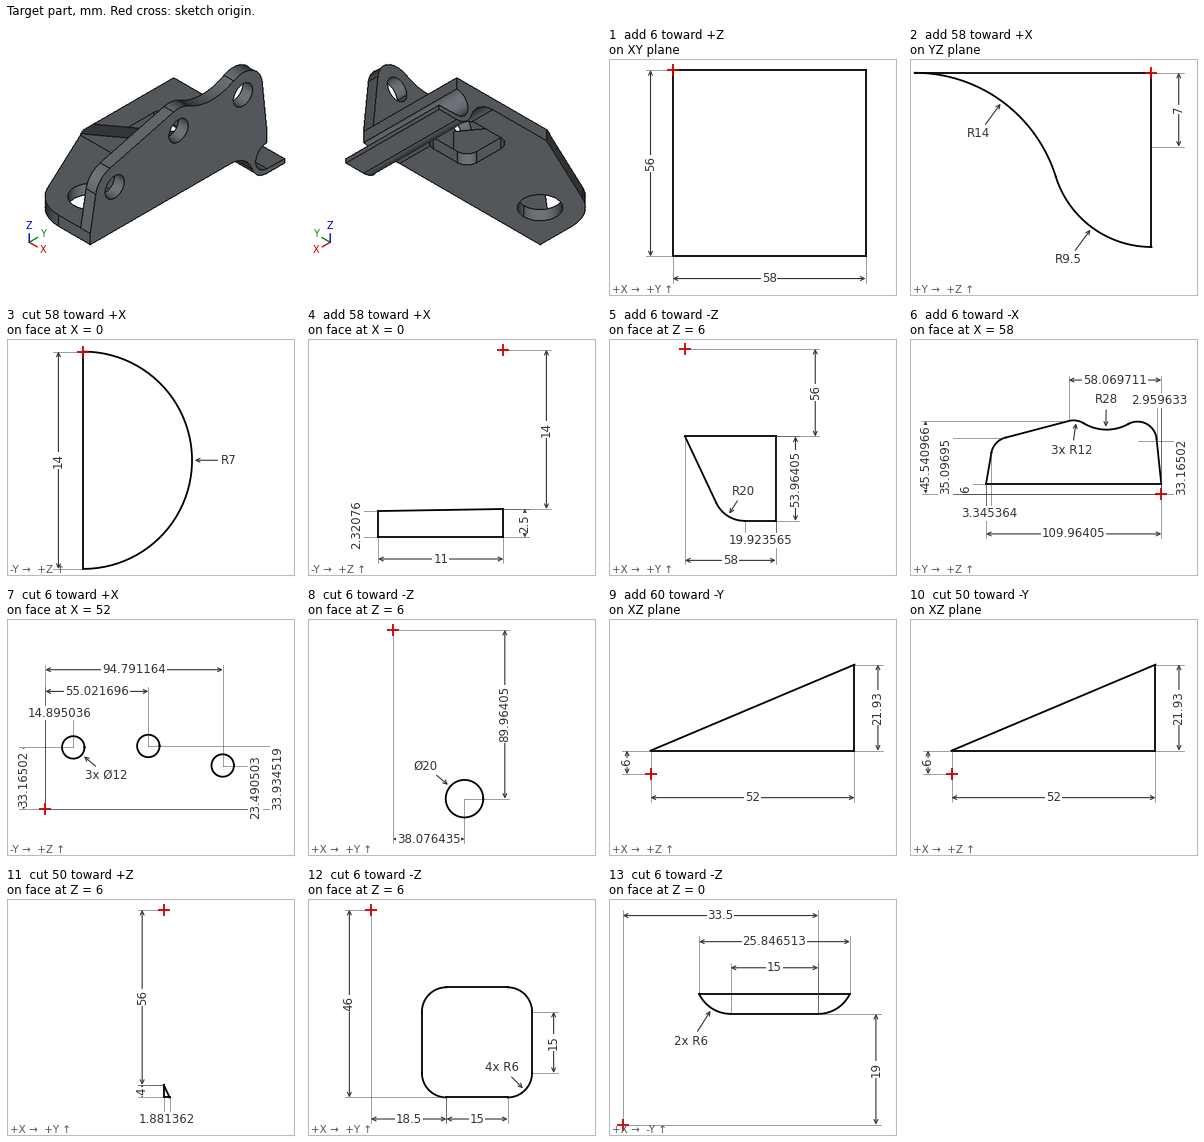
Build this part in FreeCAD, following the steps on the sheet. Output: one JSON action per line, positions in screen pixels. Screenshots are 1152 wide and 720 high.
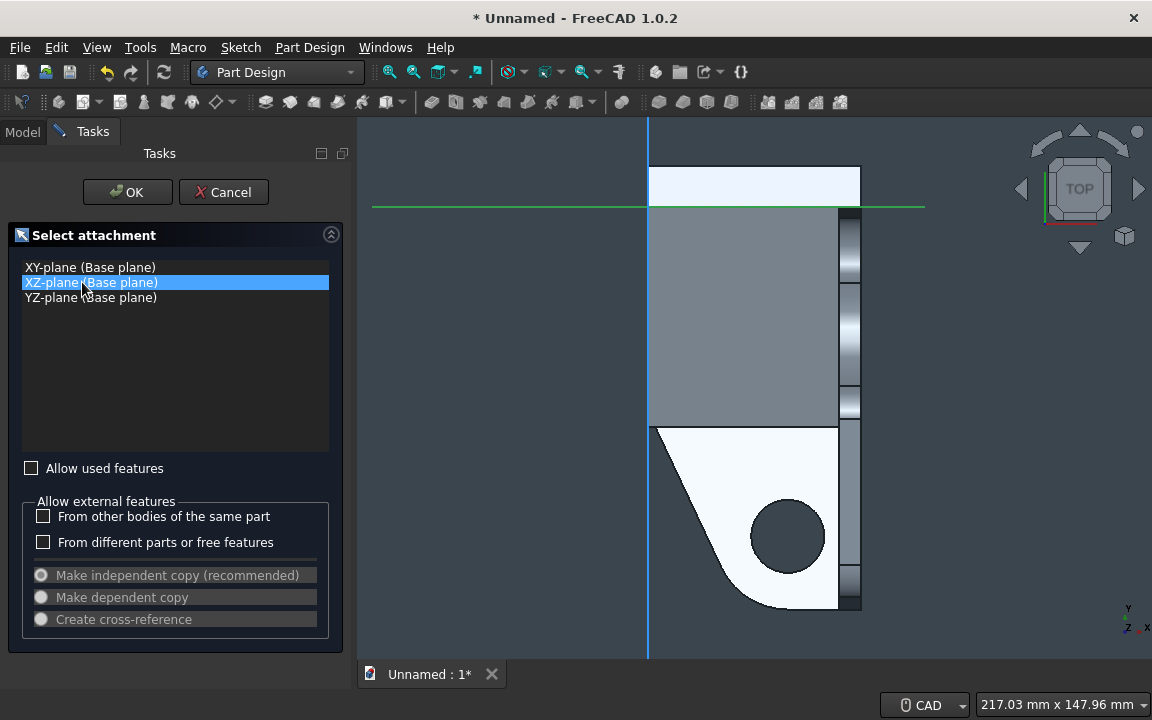
{"action": "left_click", "coordinate": [128, 192]}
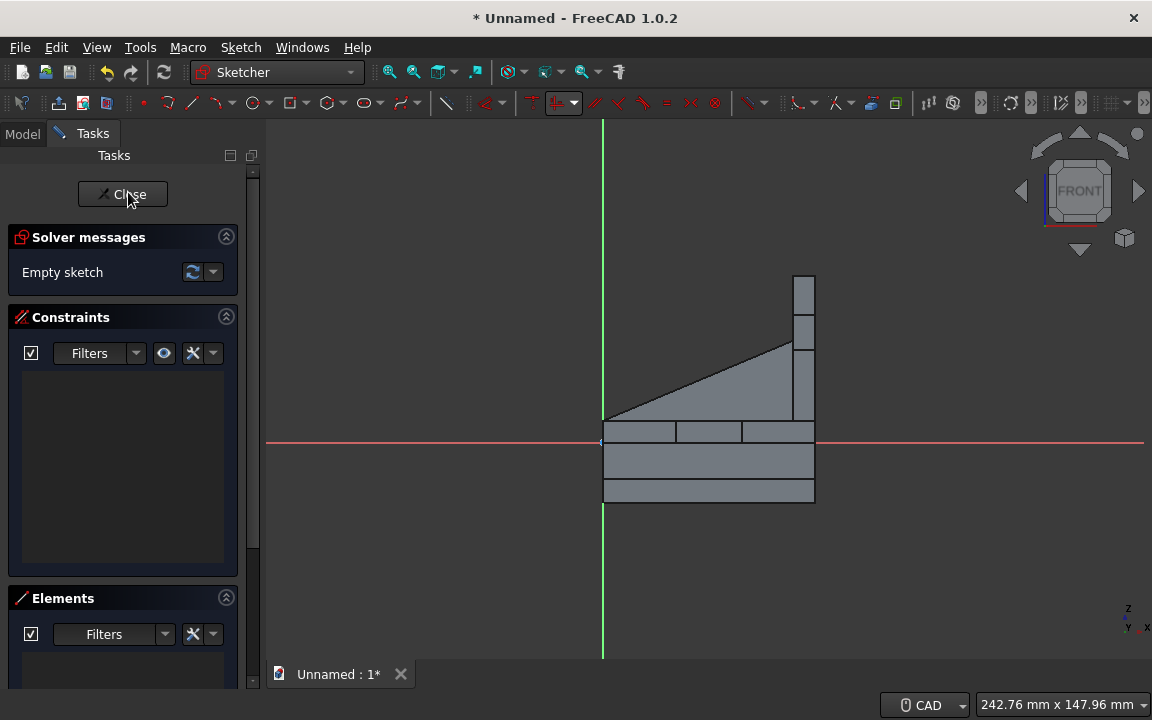
{"action": "left_click", "coordinate": [108, 104]}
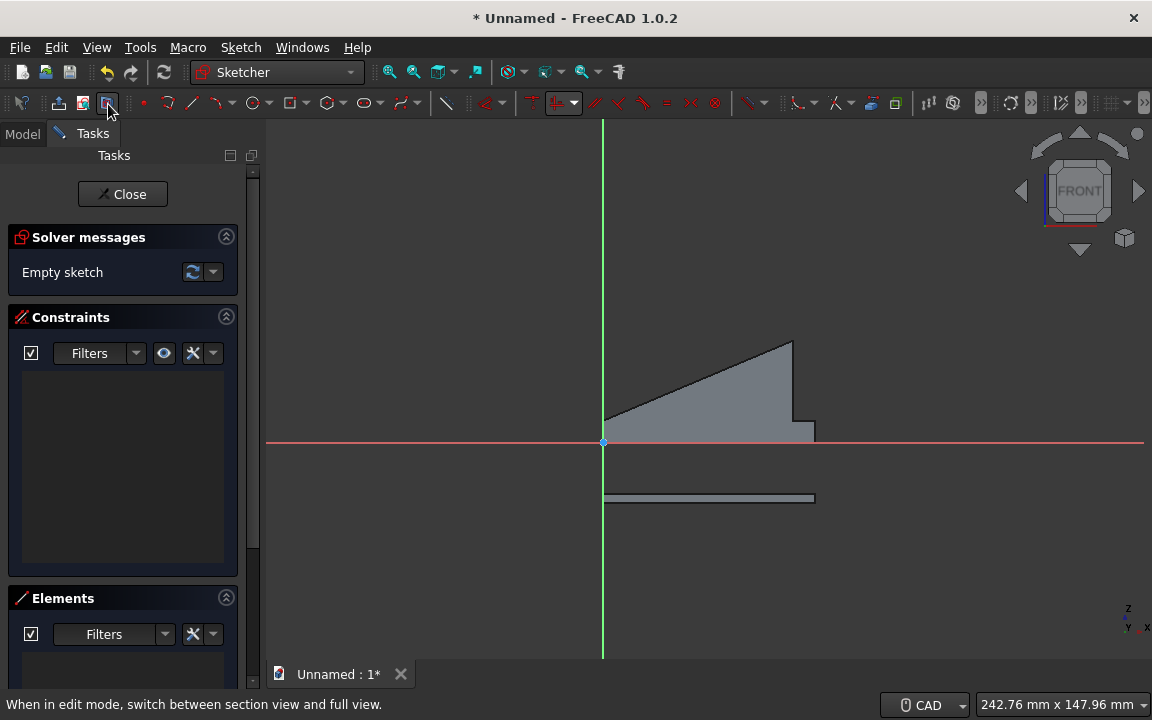
{"action": "scroll", "coordinate": [732, 393], "scroll_direction": "up", "scroll_amount": 5}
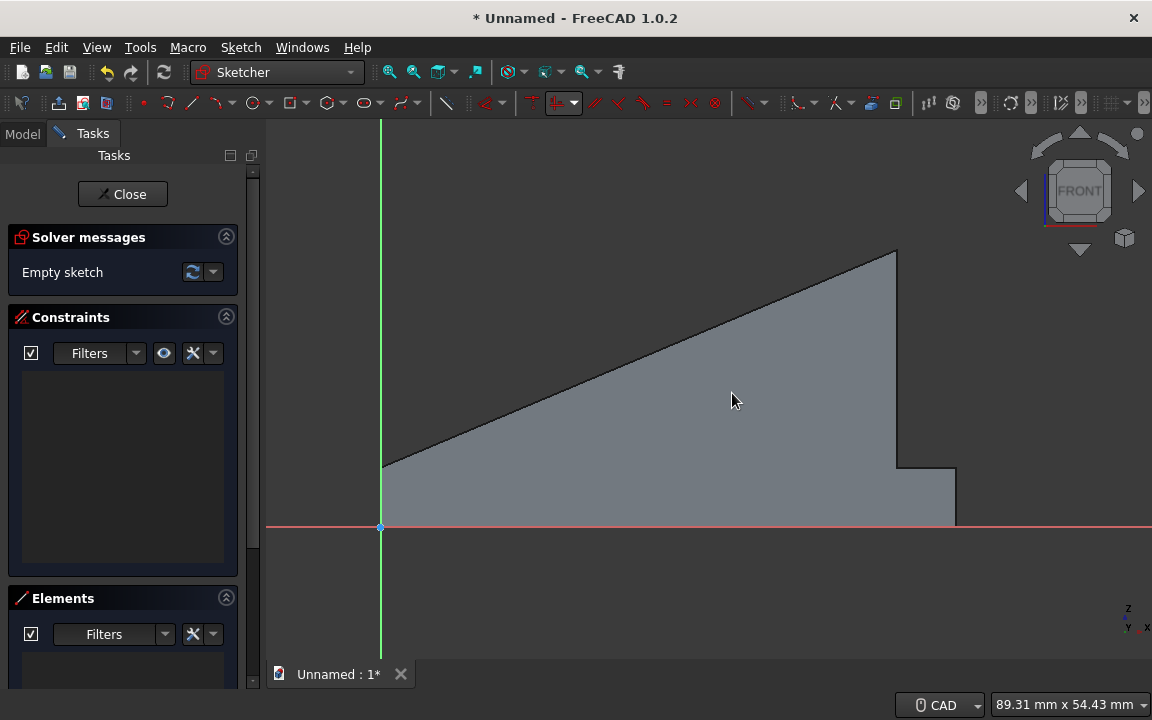
{"action": "left_click", "coordinate": [168, 104]}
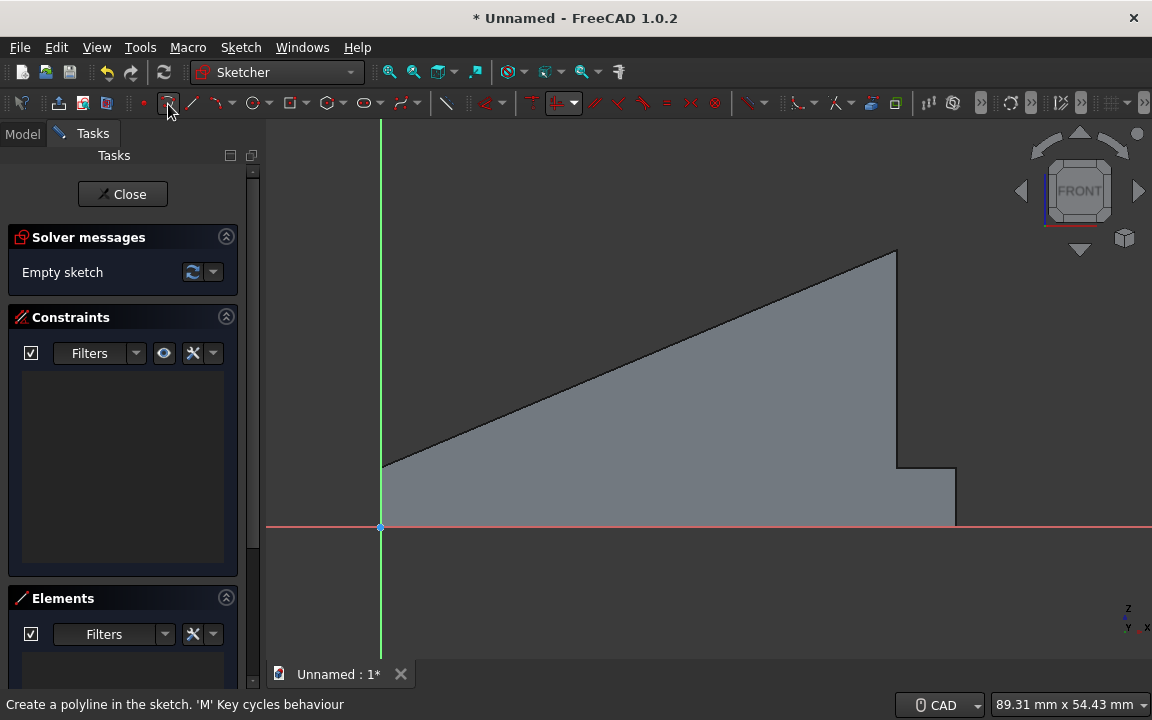
{"action": "left_click", "coordinate": [381, 468]}
{"action": "left_click", "coordinate": [897, 250]}
{"action": "left_click", "coordinate": [897, 468]}
{"action": "left_click", "coordinate": [381, 469]}
{"action": "key", "text": "Escape"}
{"action": "key", "text": "Escape"}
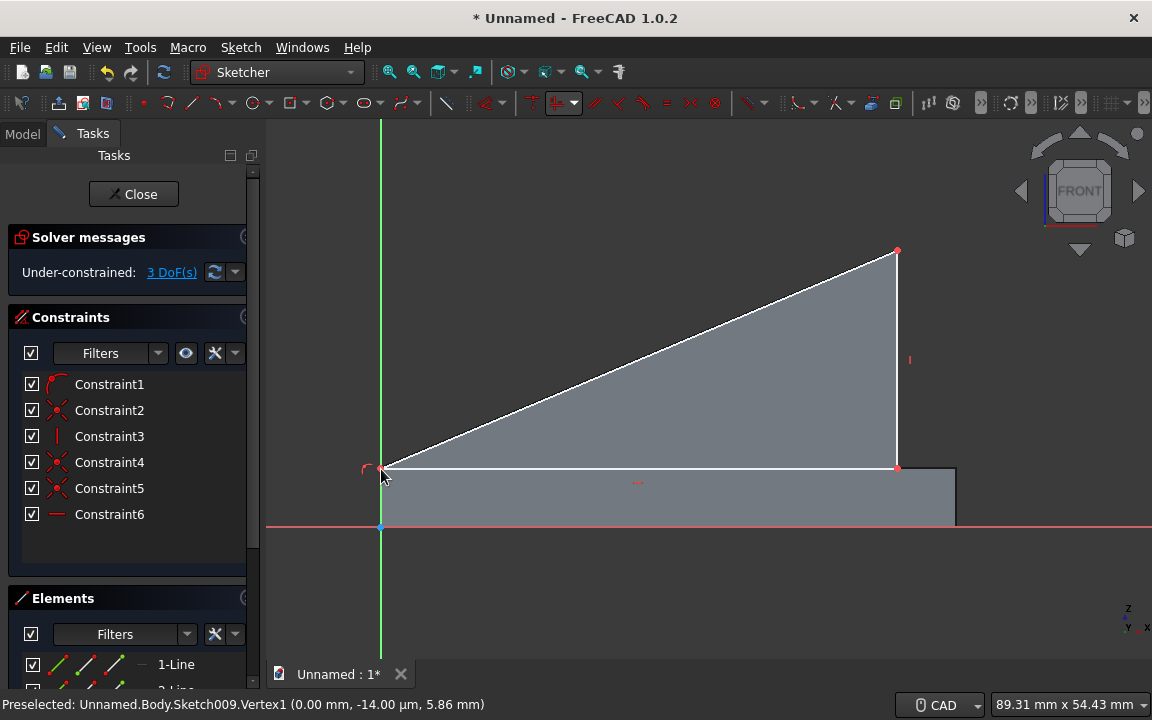
{"action": "left_click", "coordinate": [486, 104]}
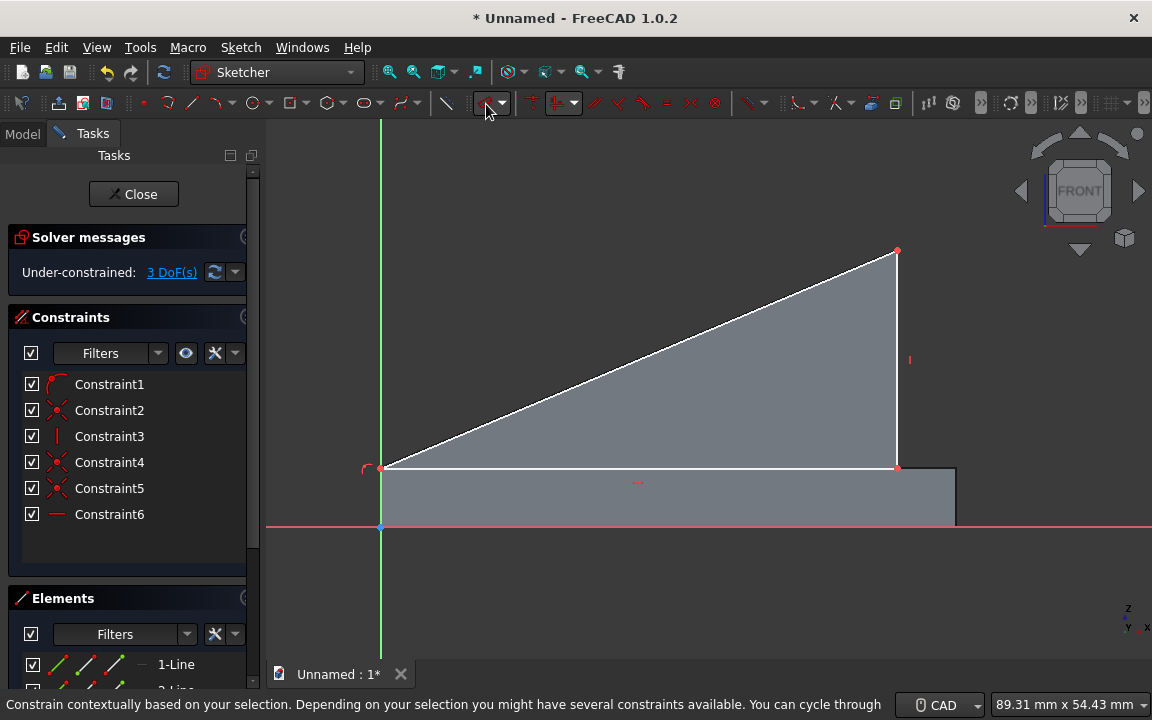
{"action": "left_click", "coordinate": [742, 469]}
{"action": "left_click", "coordinate": [639, 503]}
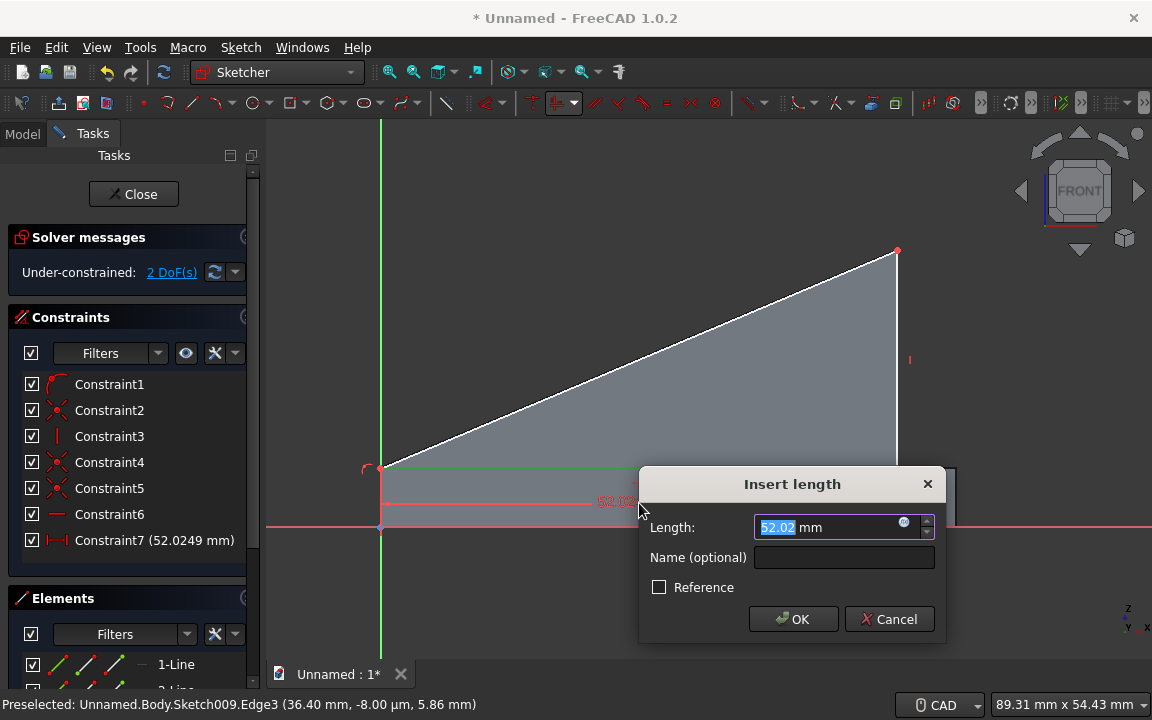
{"action": "type", "text": "52"}
{"action": "key", "text": "Return"}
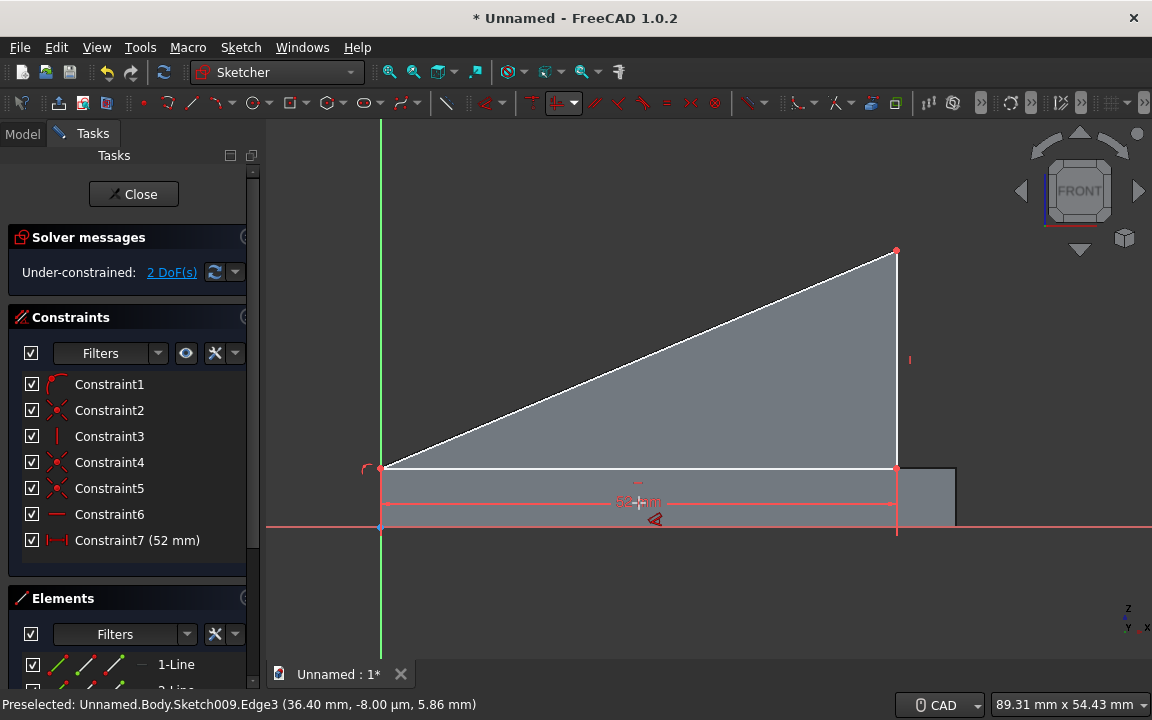
{"action": "left_click", "coordinate": [381, 469]}
{"action": "left_click", "coordinate": [347, 498]}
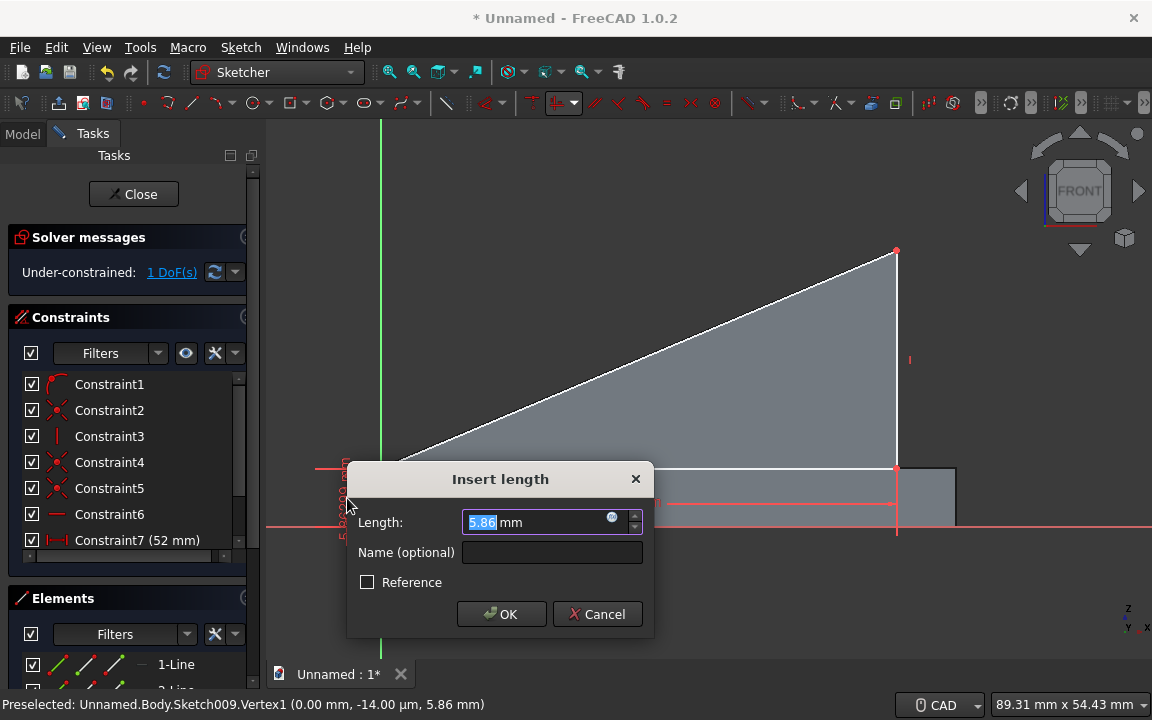
{"action": "type", "text": "6"}
{"action": "key", "text": "Return"}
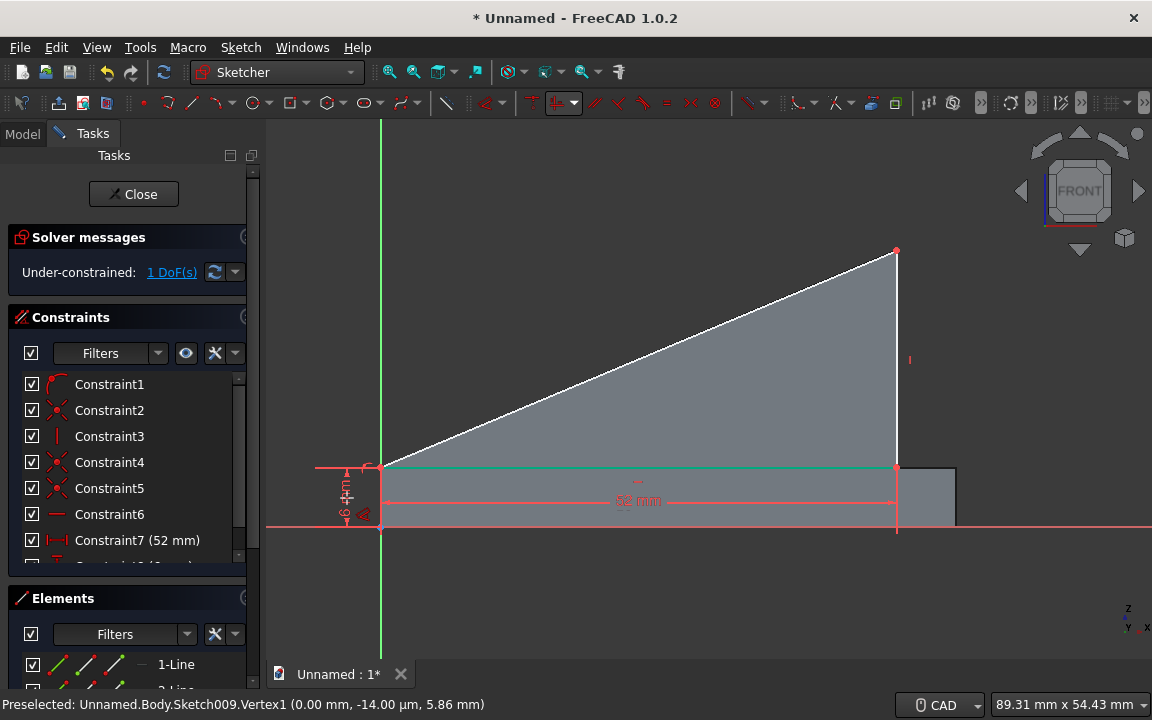
{"action": "left_click", "coordinate": [897, 316]}
{"action": "left_click", "coordinate": [931, 359]}